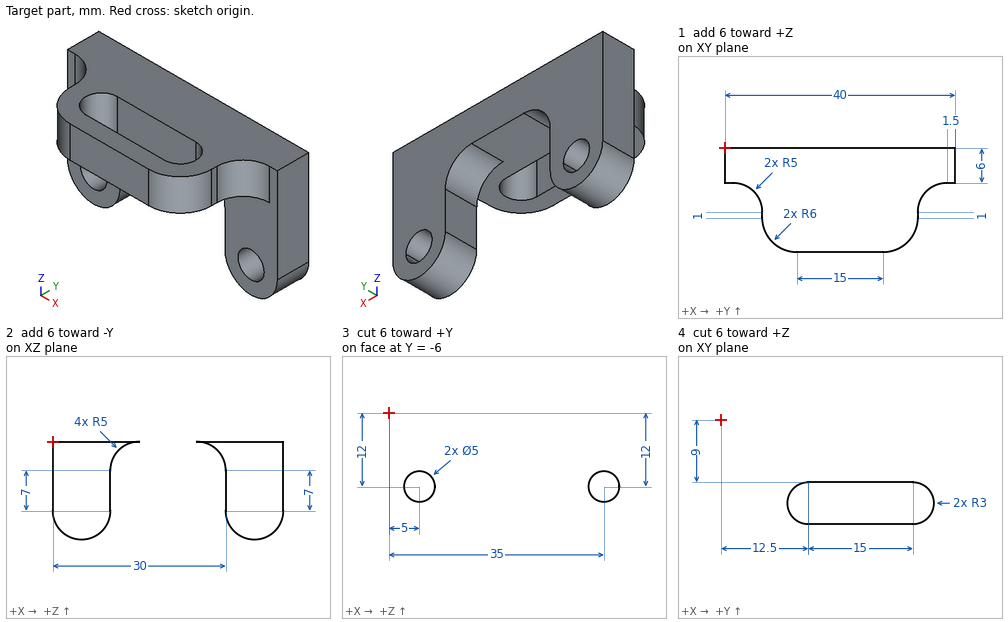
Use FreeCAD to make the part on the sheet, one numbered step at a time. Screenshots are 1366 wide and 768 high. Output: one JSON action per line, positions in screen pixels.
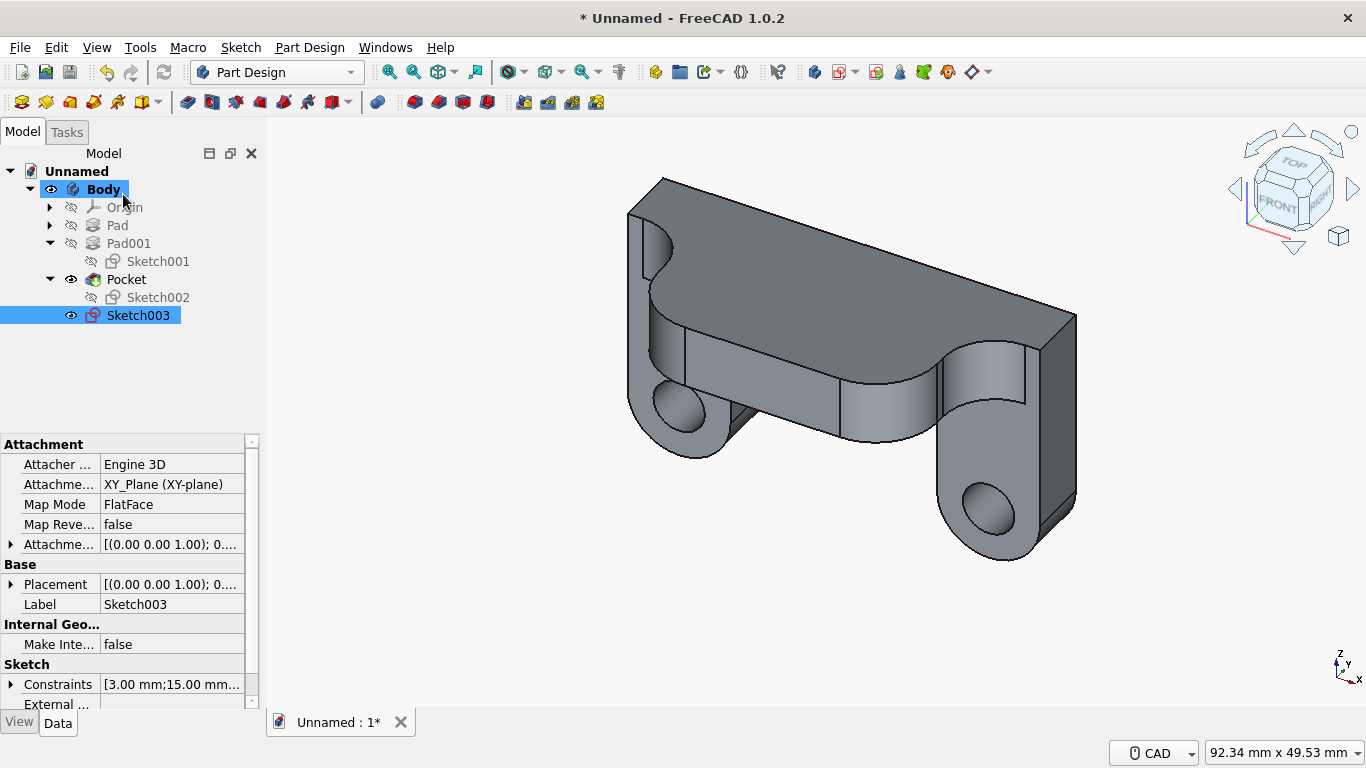
{"action": "left_click", "coordinate": [188, 102]}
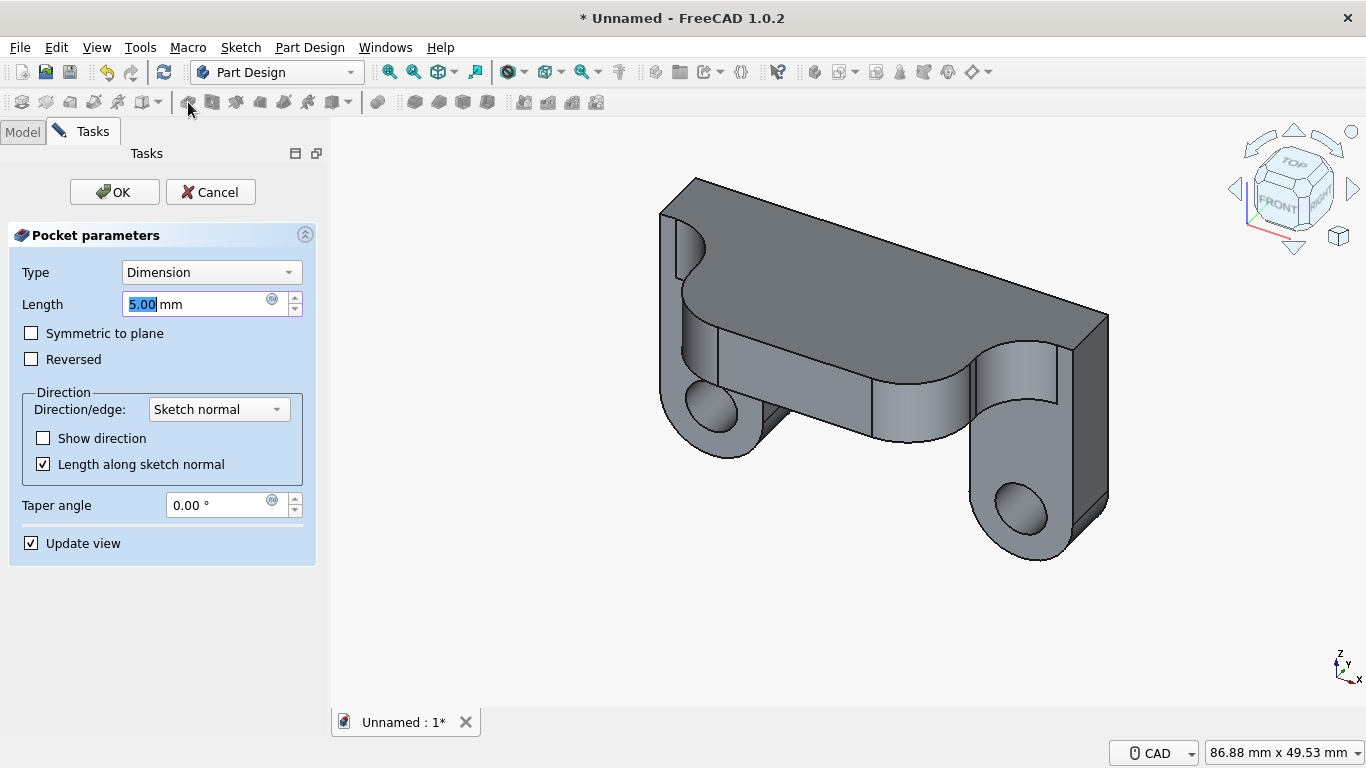
{"action": "type", "text": "6"}
{"action": "key", "text": "Tab"}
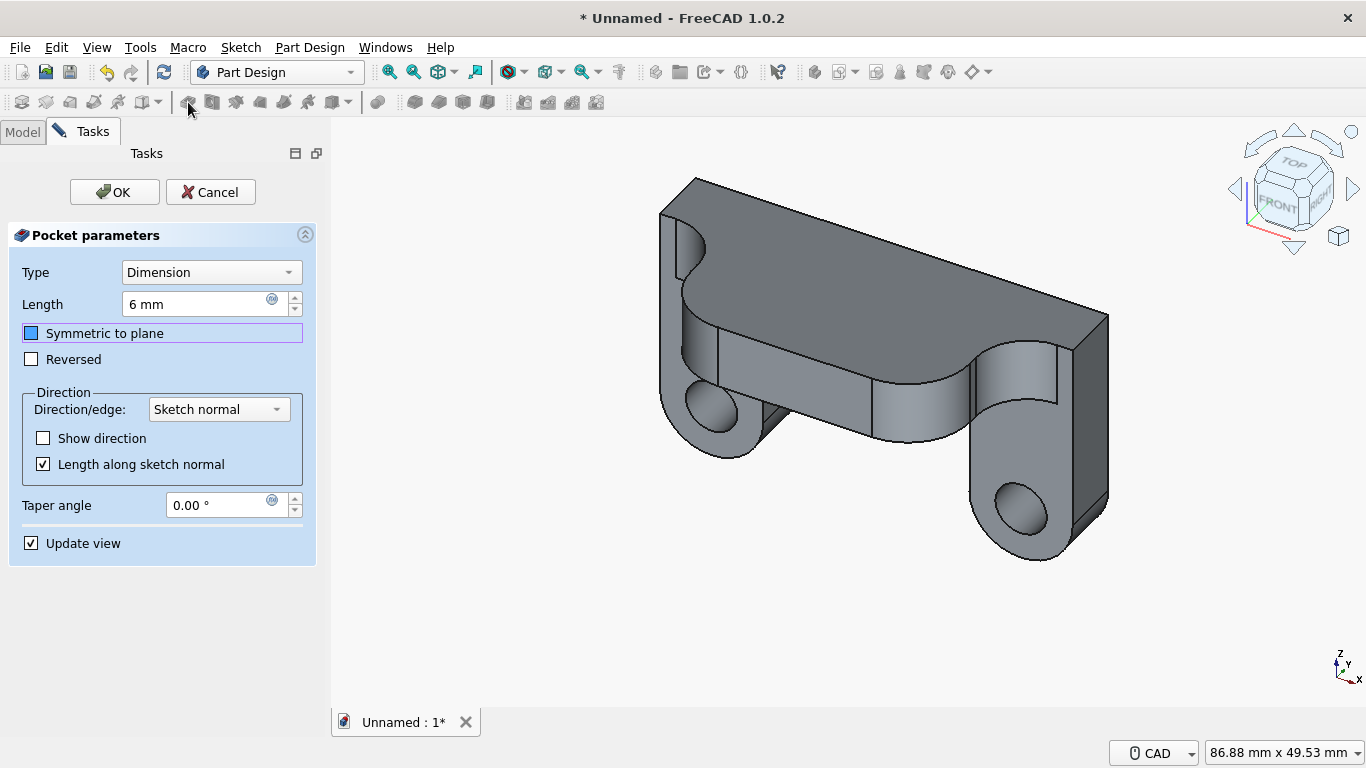
{"action": "left_click", "coordinate": [30, 359]}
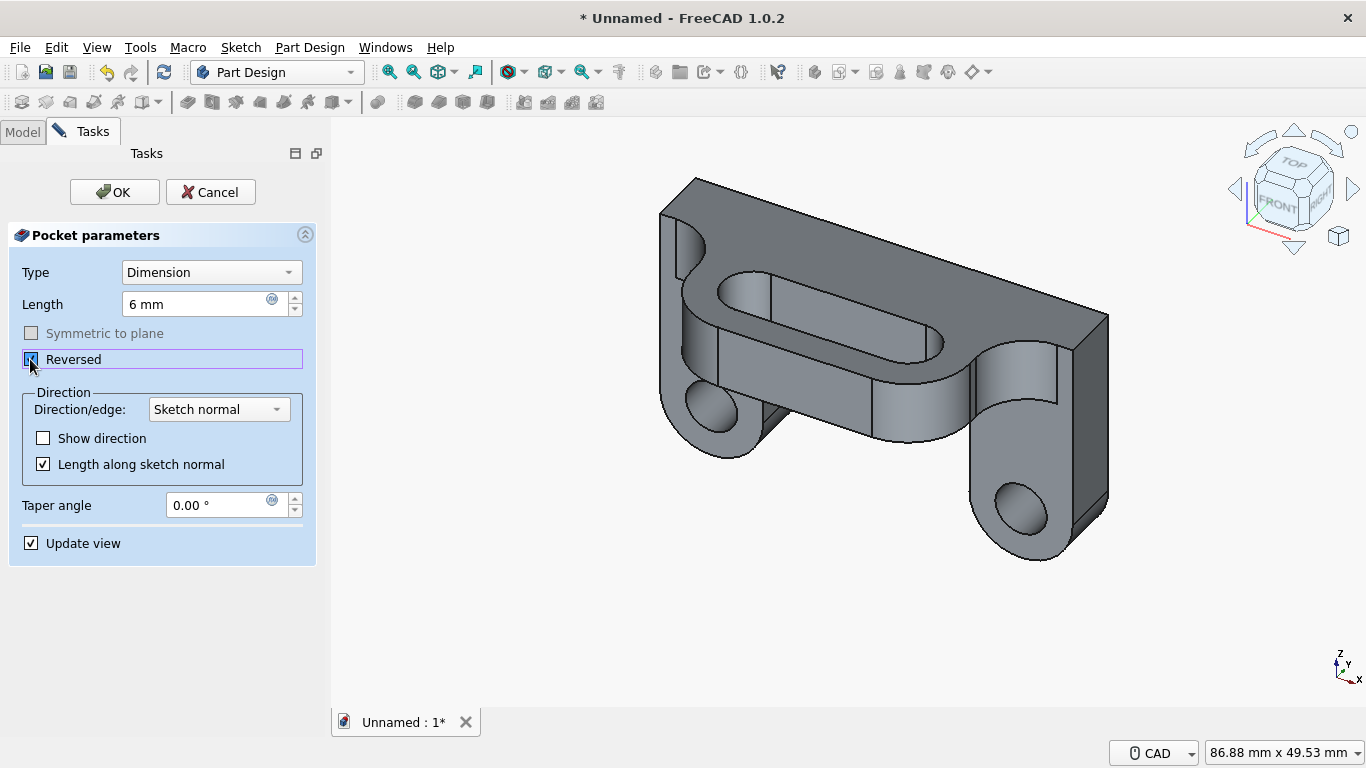
{"action": "left_click", "coordinate": [115, 192]}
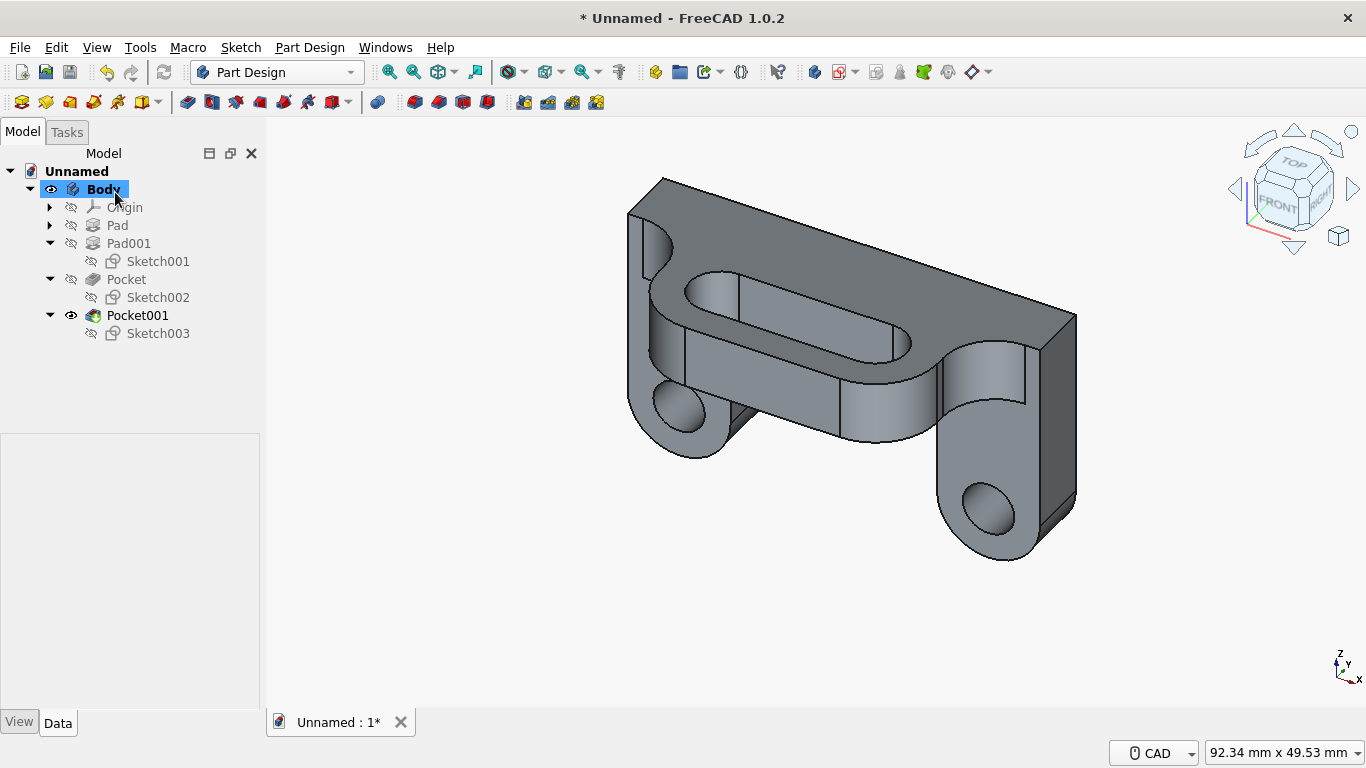
{"action": "key", "text": "0"}